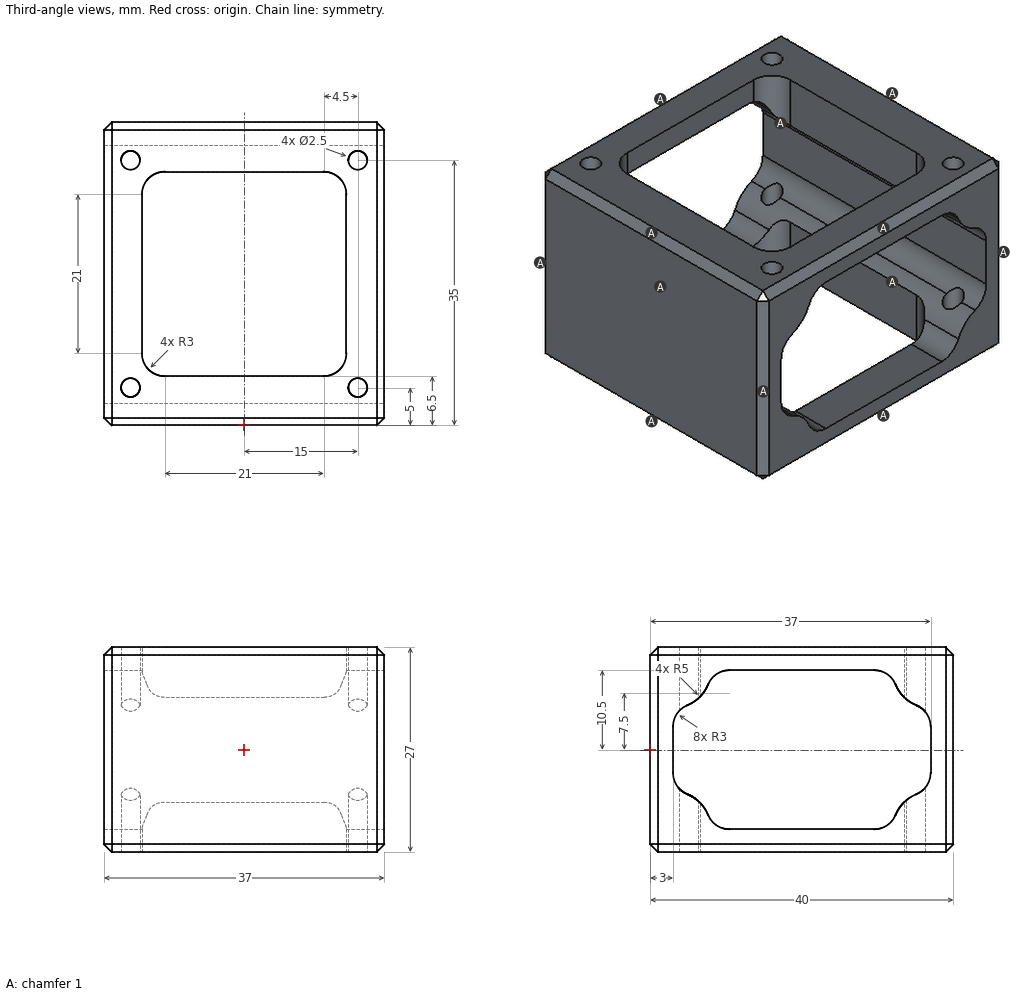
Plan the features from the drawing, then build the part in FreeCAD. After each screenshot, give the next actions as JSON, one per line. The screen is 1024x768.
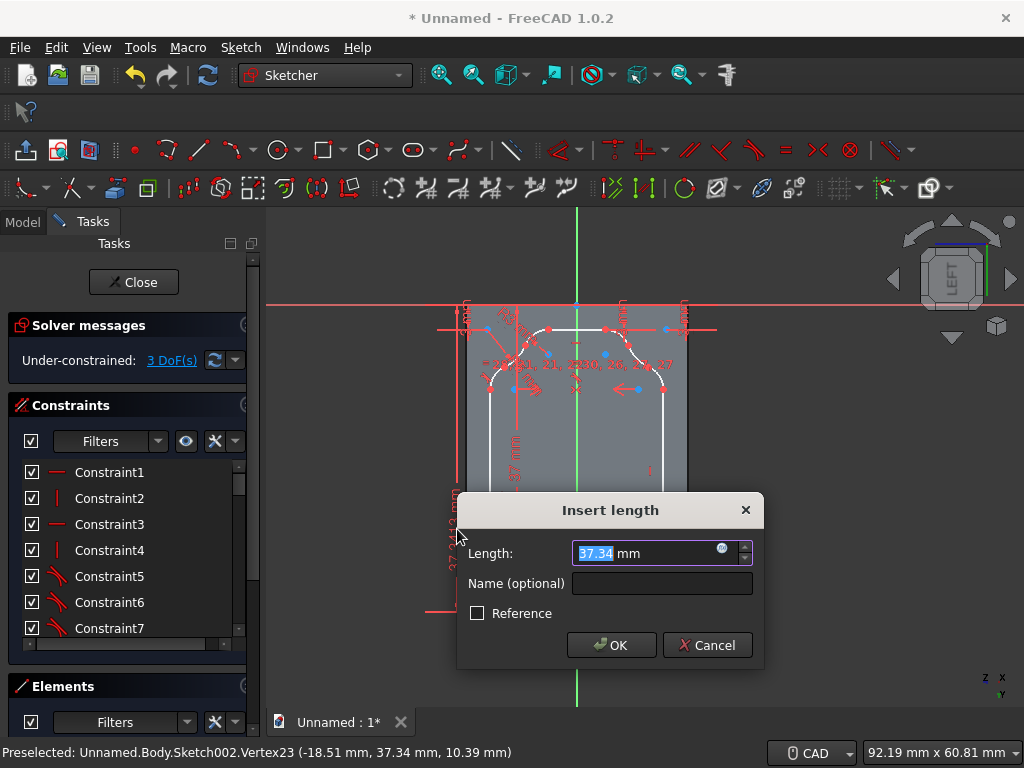
{"action": "type", "text": "37"}
{"action": "key", "text": "Return"}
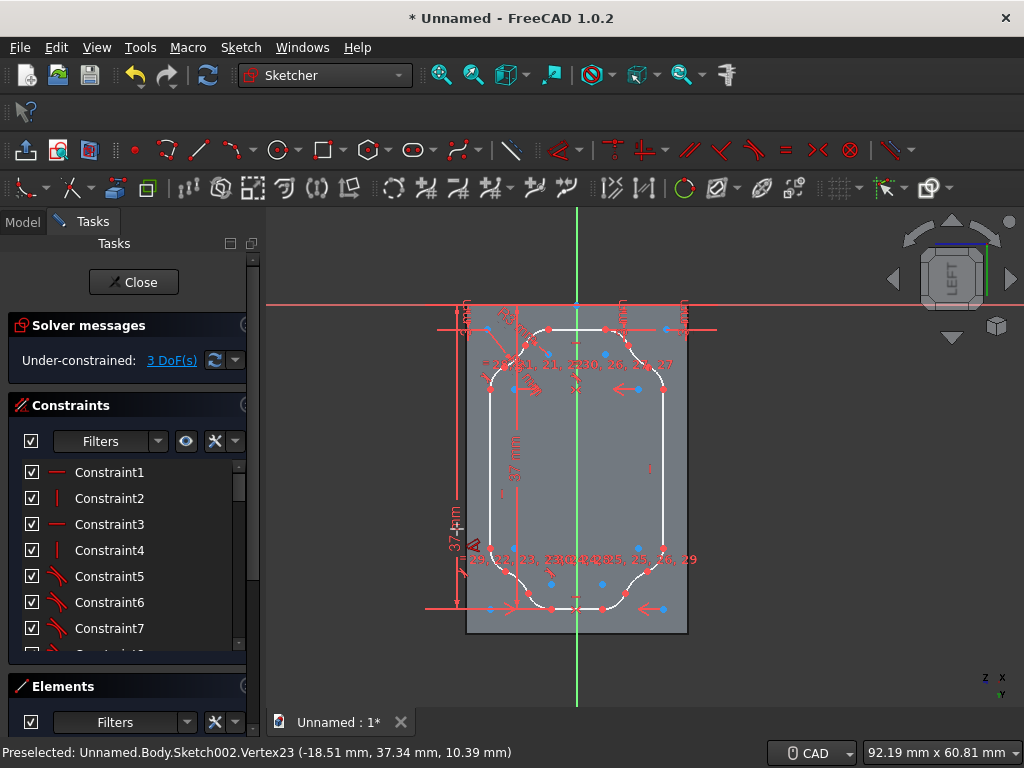
{"action": "left_click", "coordinate": [515, 389]}
{"action": "left_click", "coordinate": [546, 271]}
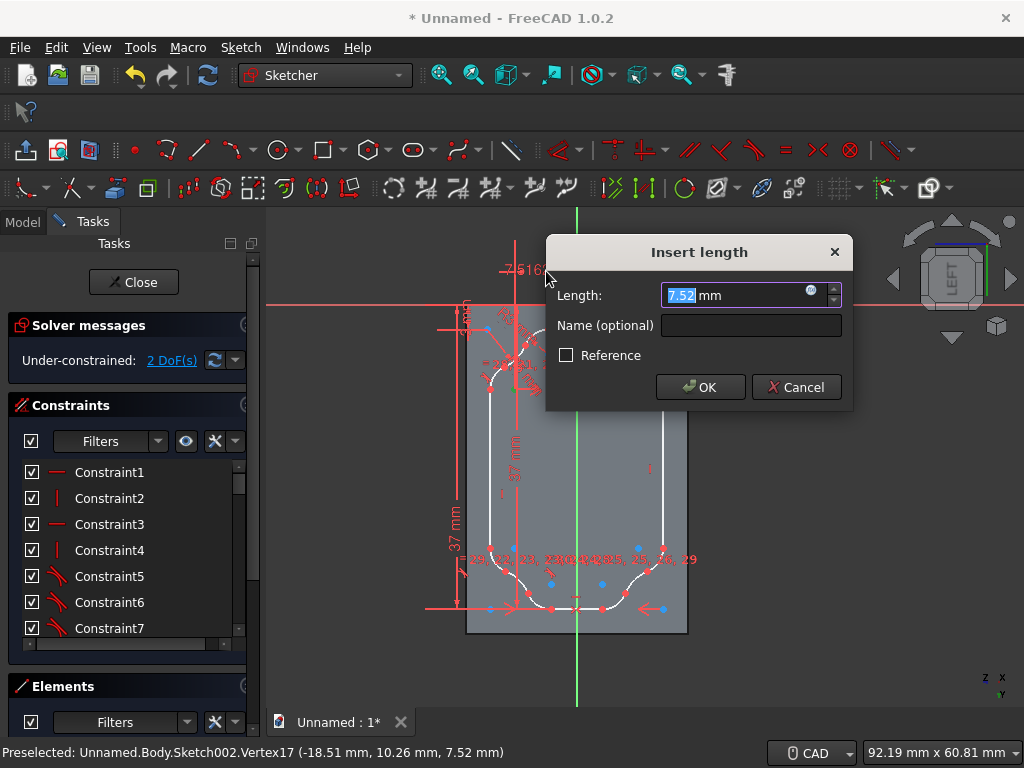
{"action": "type", "text": "7.5"}
{"action": "key", "text": "Return"}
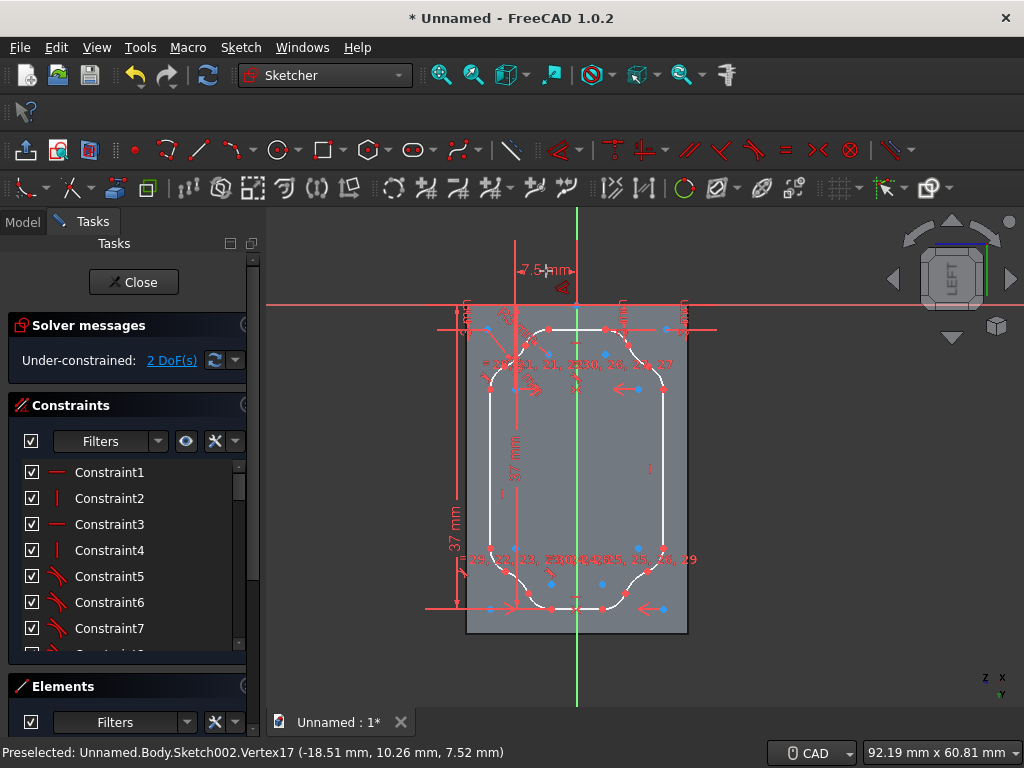
{"action": "left_click", "coordinate": [487, 330]}
{"action": "left_click", "coordinate": [532, 247]}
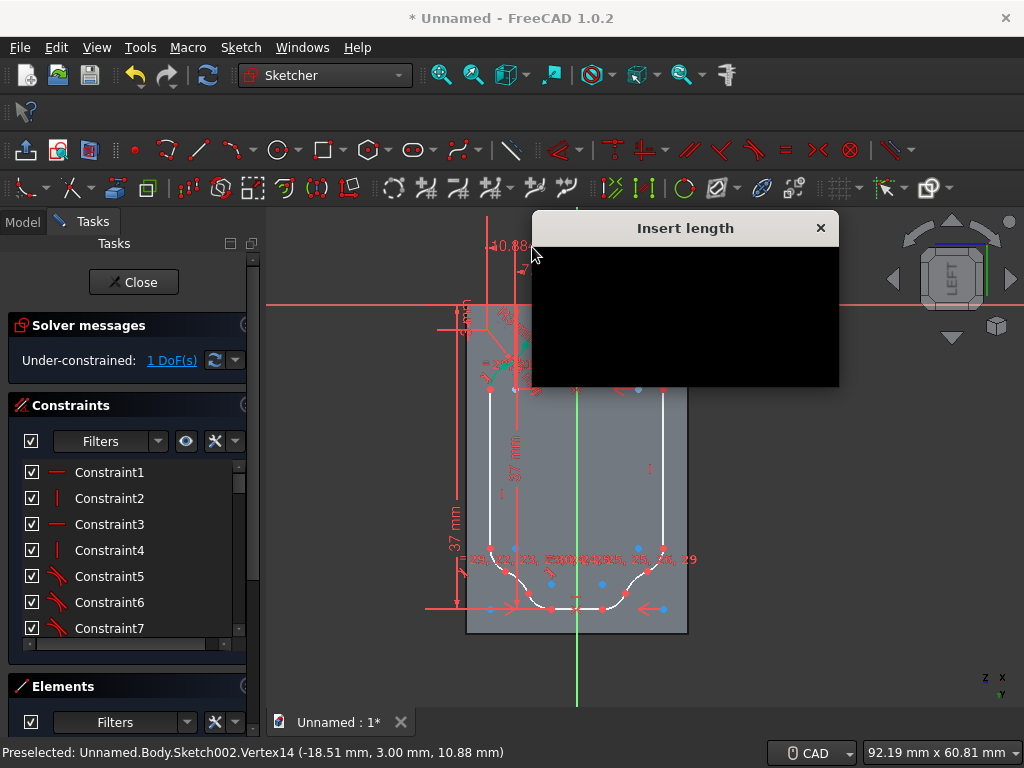
{"action": "type", "text": "10.5"}
{"action": "key", "text": "Return"}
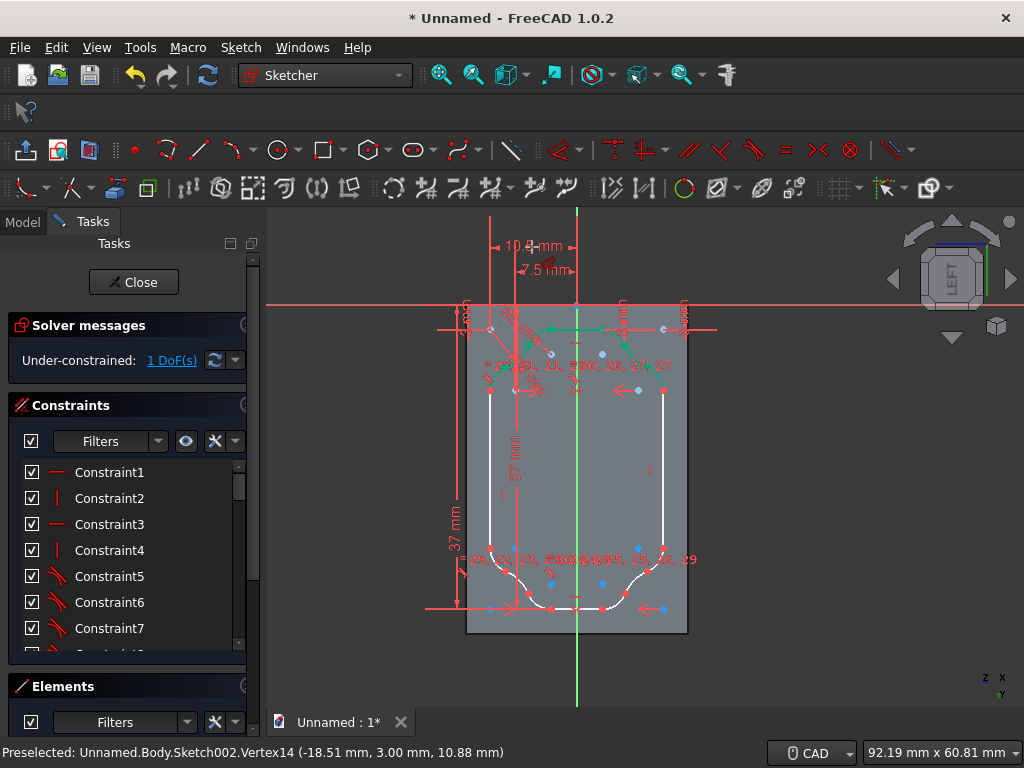
{"action": "left_click", "coordinate": [490, 609]}
{"action": "left_click", "coordinate": [533, 643]}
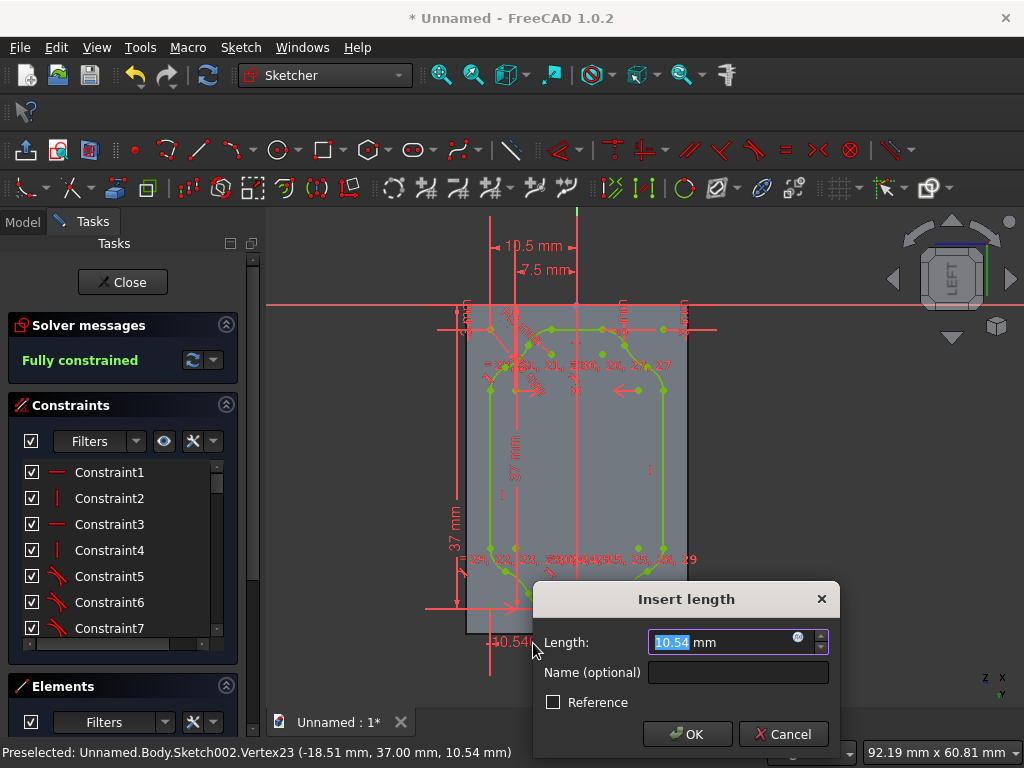
{"action": "type", "text": "10.5"}
{"action": "key", "text": "Return"}
{"action": "key", "text": "Escape"}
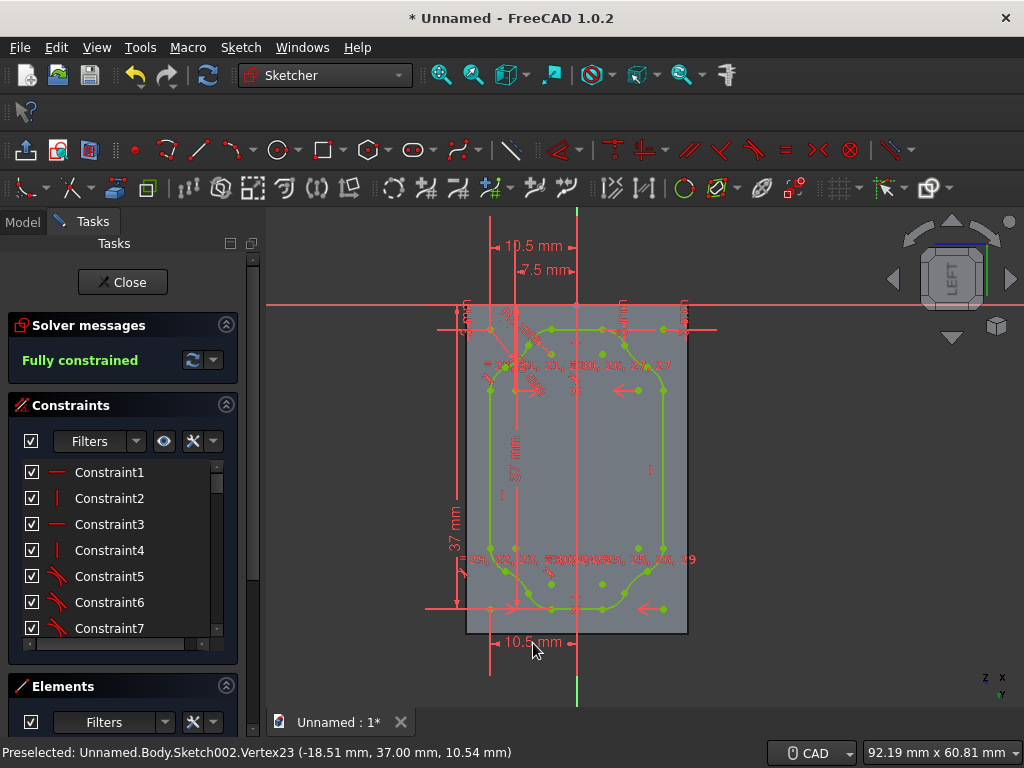
{"action": "left_click", "coordinate": [123, 282]}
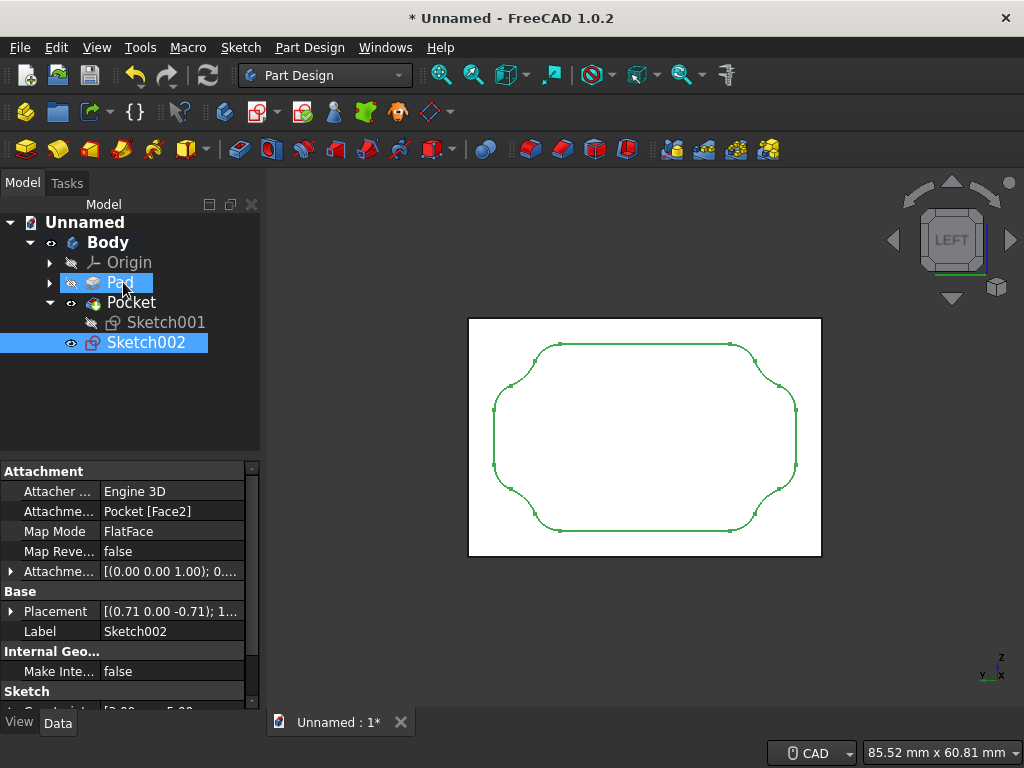
{"action": "left_click", "coordinate": [240, 150]}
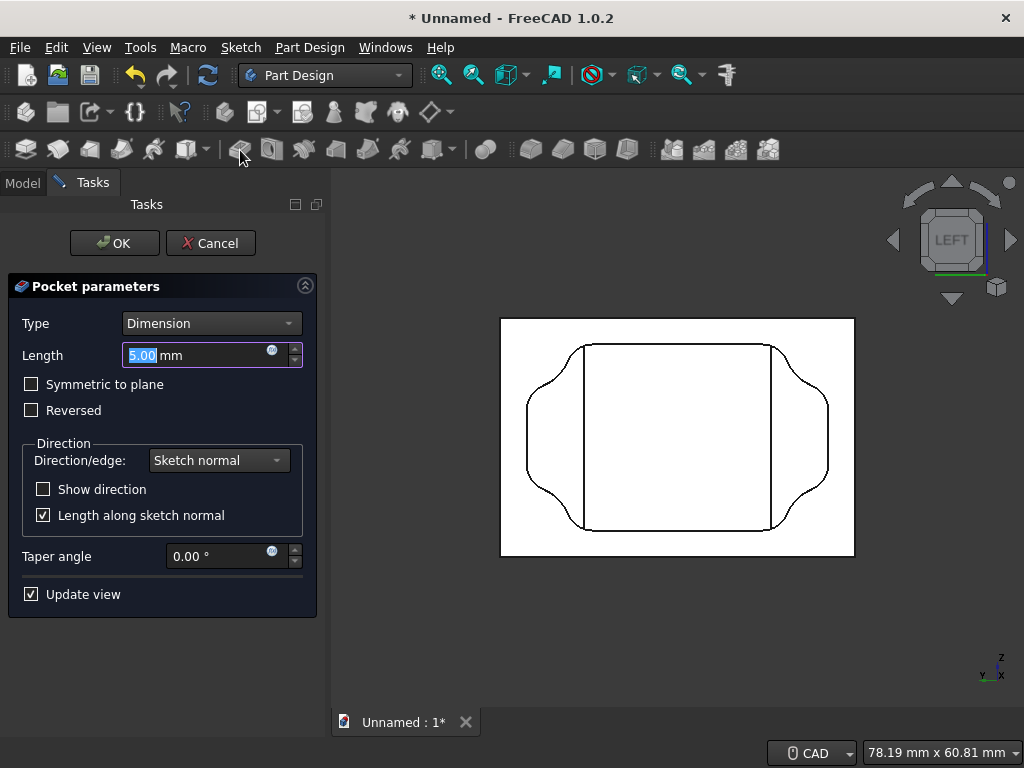
{"action": "left_click", "coordinate": [212, 324]}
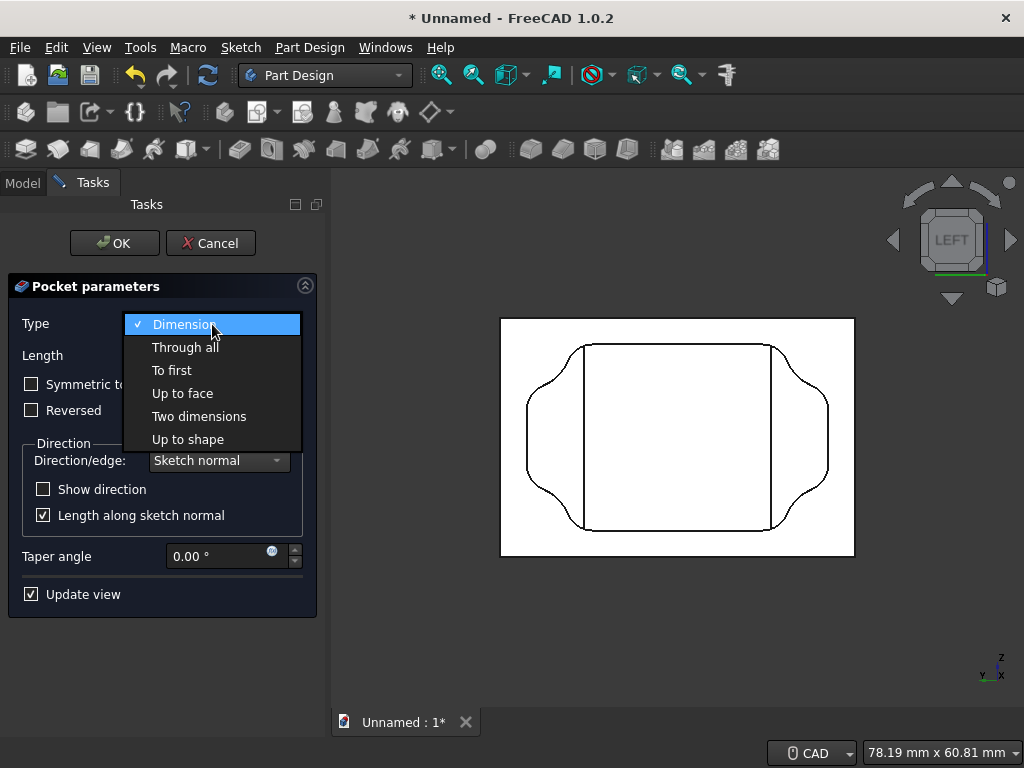
{"action": "left_click", "coordinate": [212, 348]}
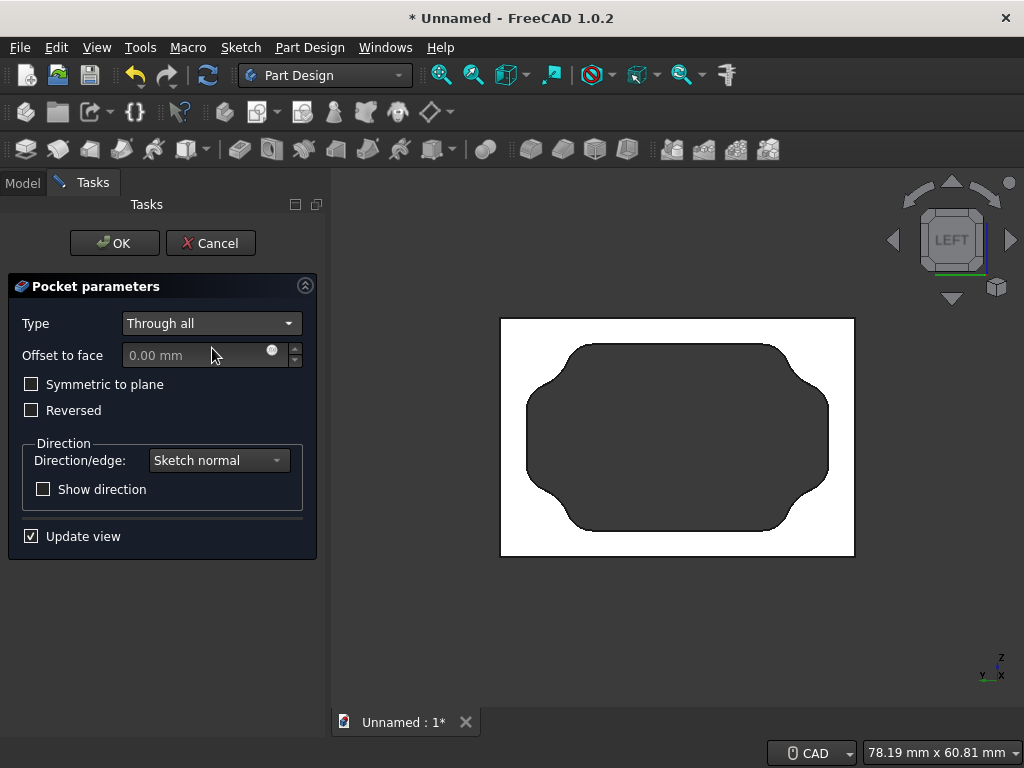
{"action": "left_click", "coordinate": [115, 243]}